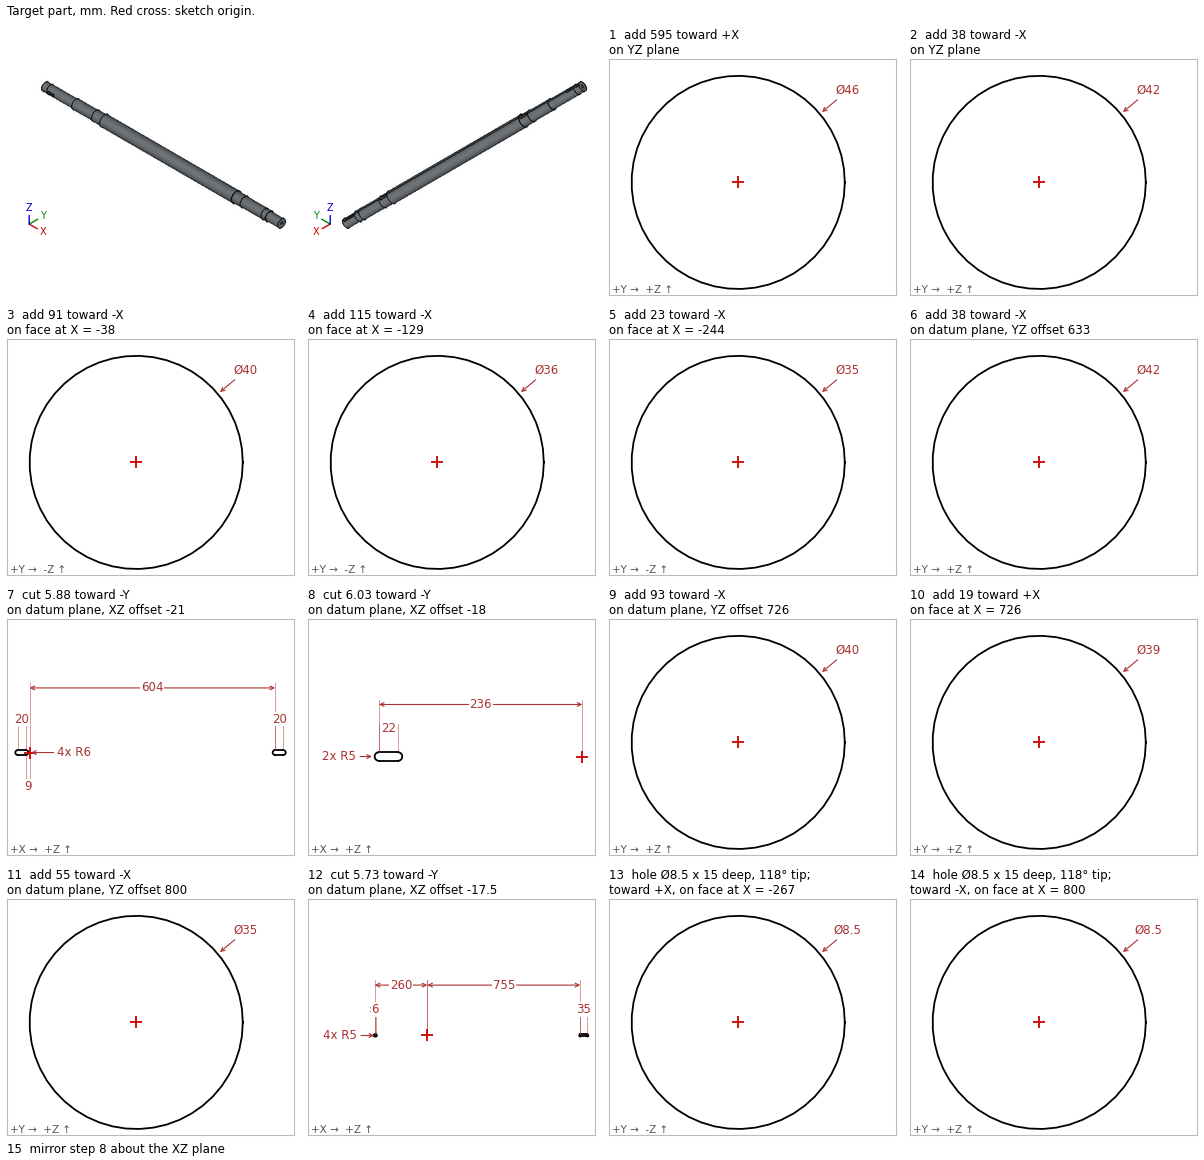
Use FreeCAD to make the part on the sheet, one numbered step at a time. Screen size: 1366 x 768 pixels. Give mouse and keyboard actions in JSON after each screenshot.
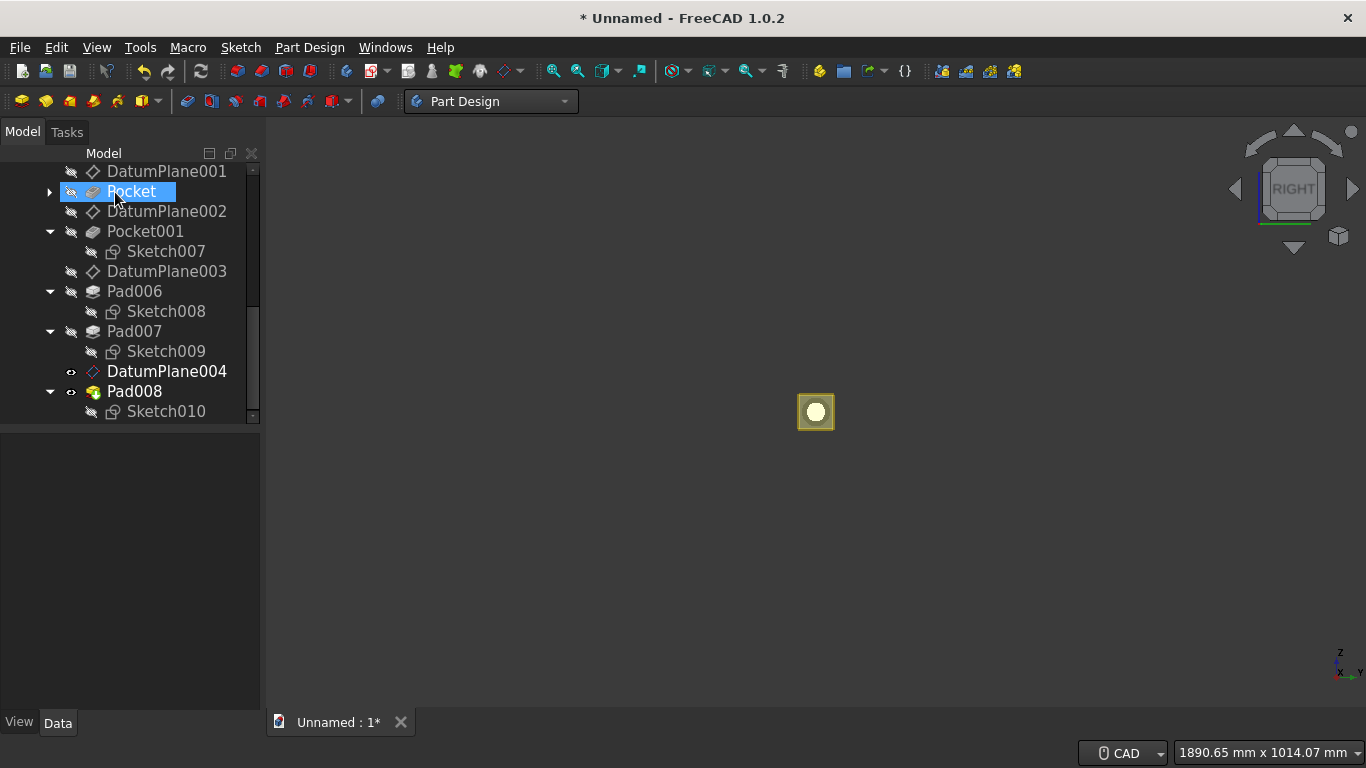
{"action": "left_click", "coordinate": [116, 372]}
{"action": "key", "text": "space"}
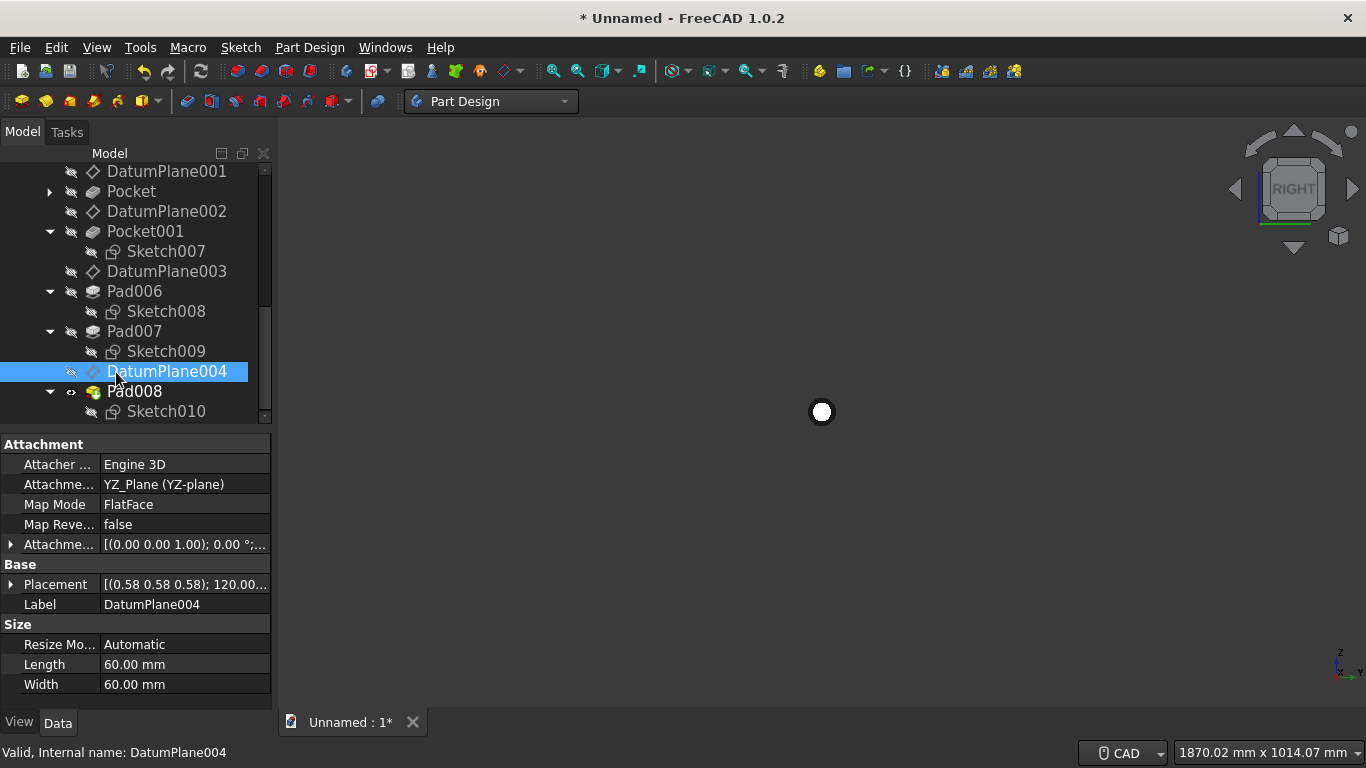
{"action": "key", "text": "v f"}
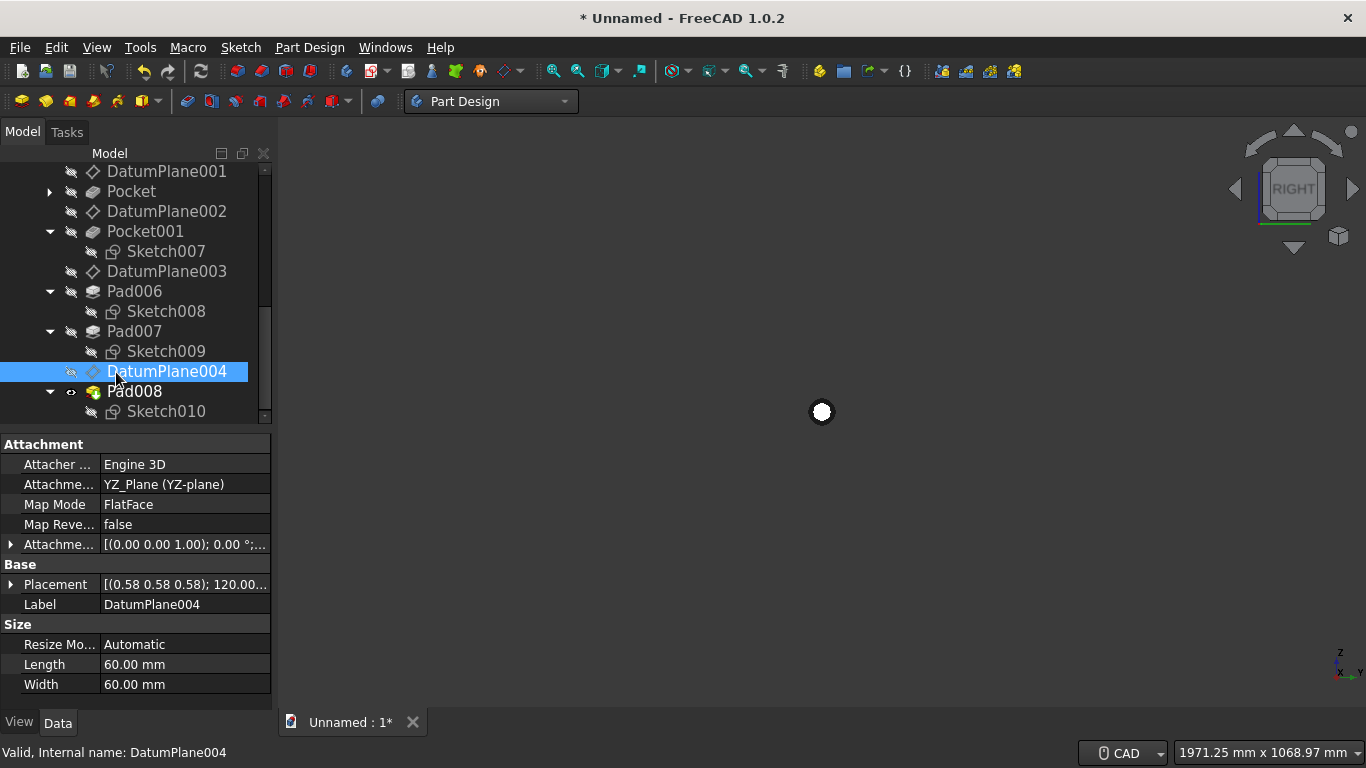
{"action": "scroll", "coordinate": [140, 287], "scroll_direction": "down", "scroll_amount": 3}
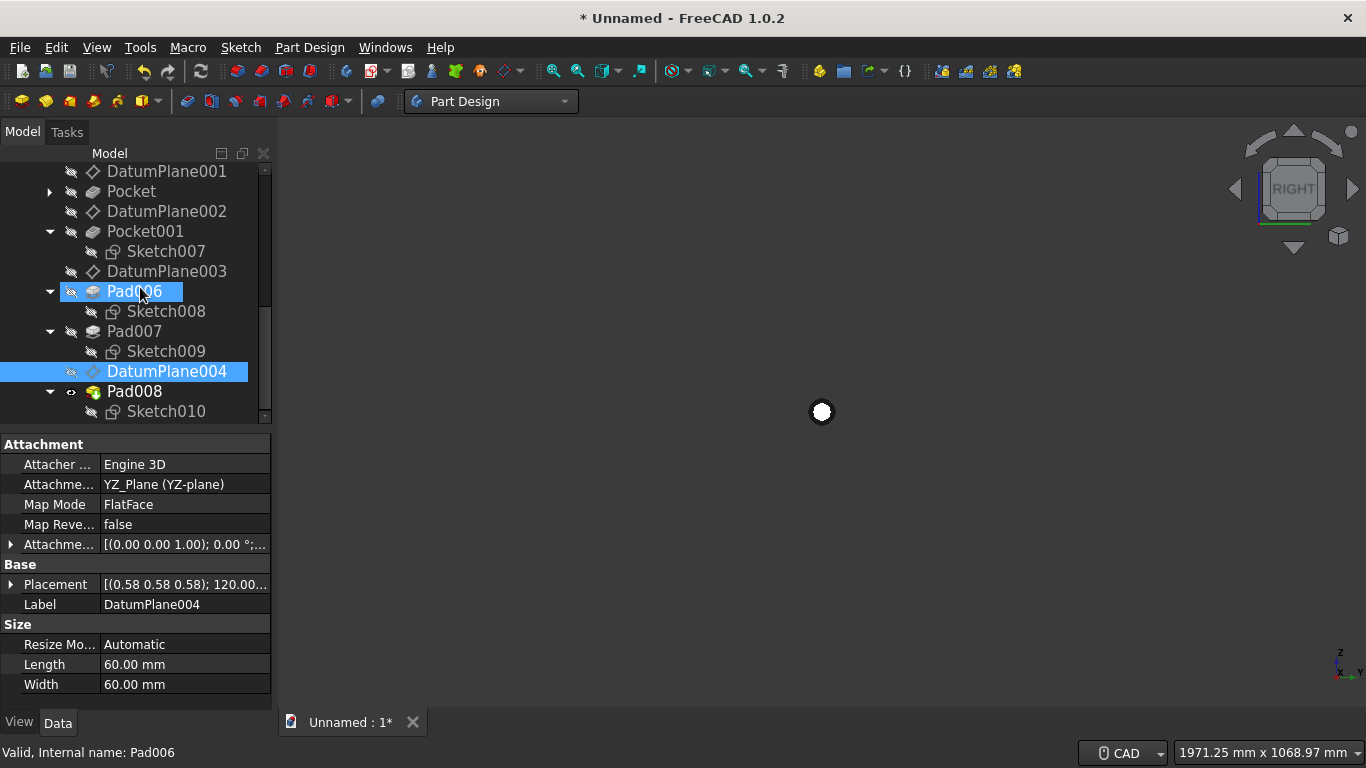
{"action": "scroll", "coordinate": [140, 287], "scroll_direction": "up", "scroll_amount": 15}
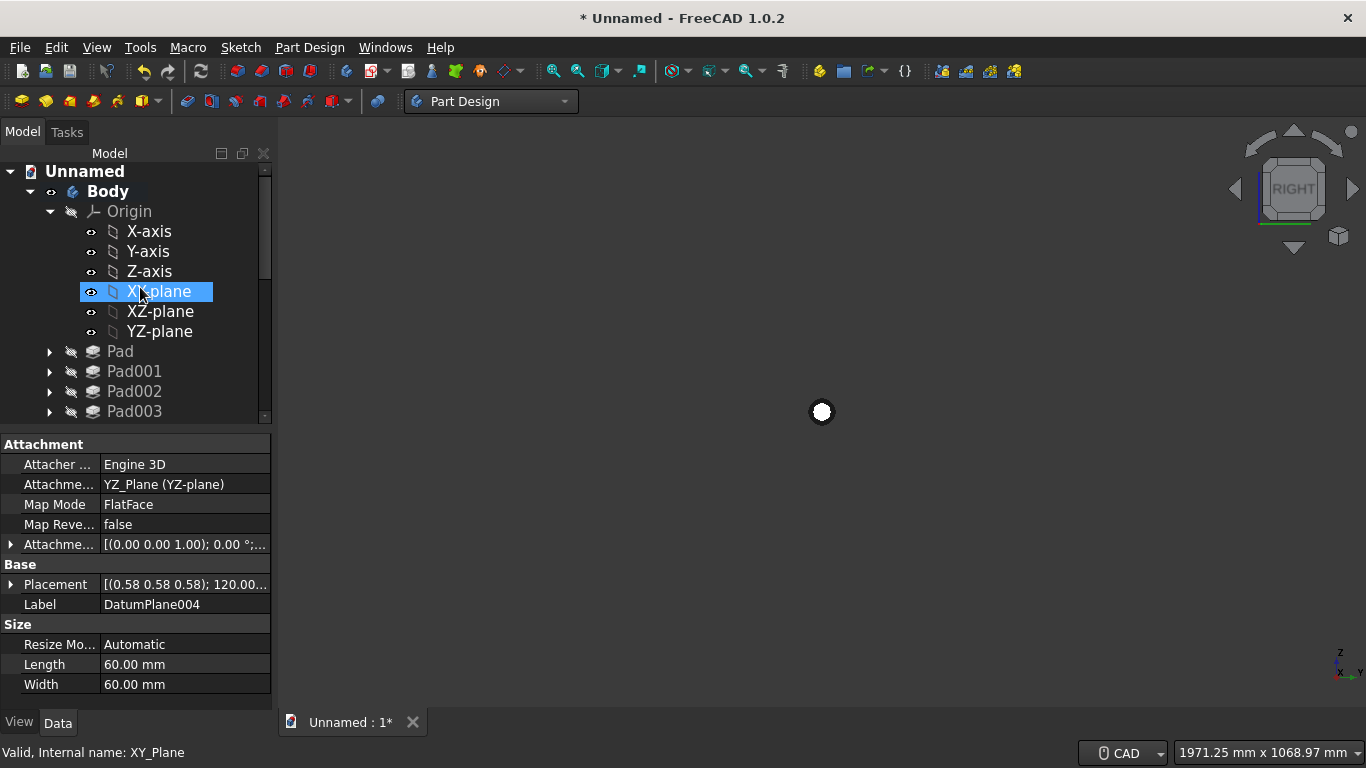
{"action": "left_click", "coordinate": [136, 312]}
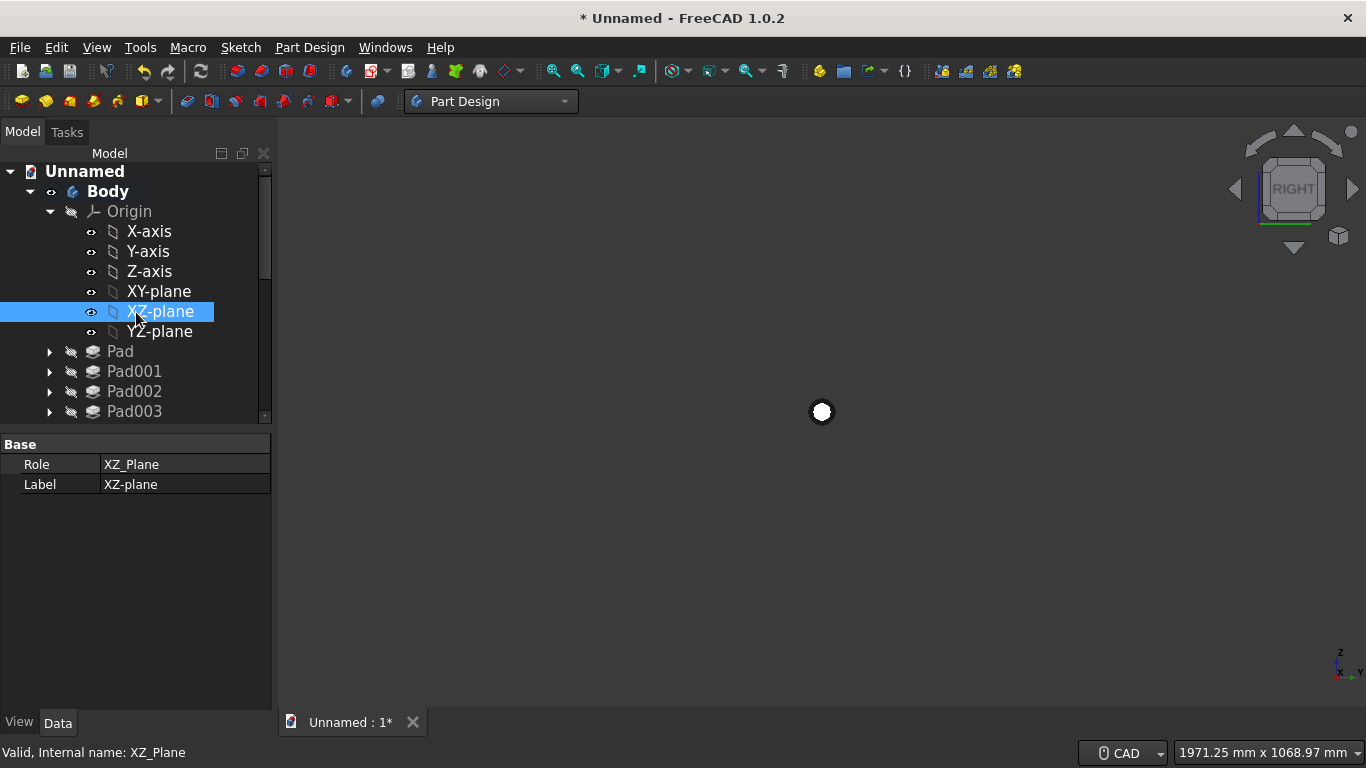
{"action": "left_click", "coordinate": [504, 72]}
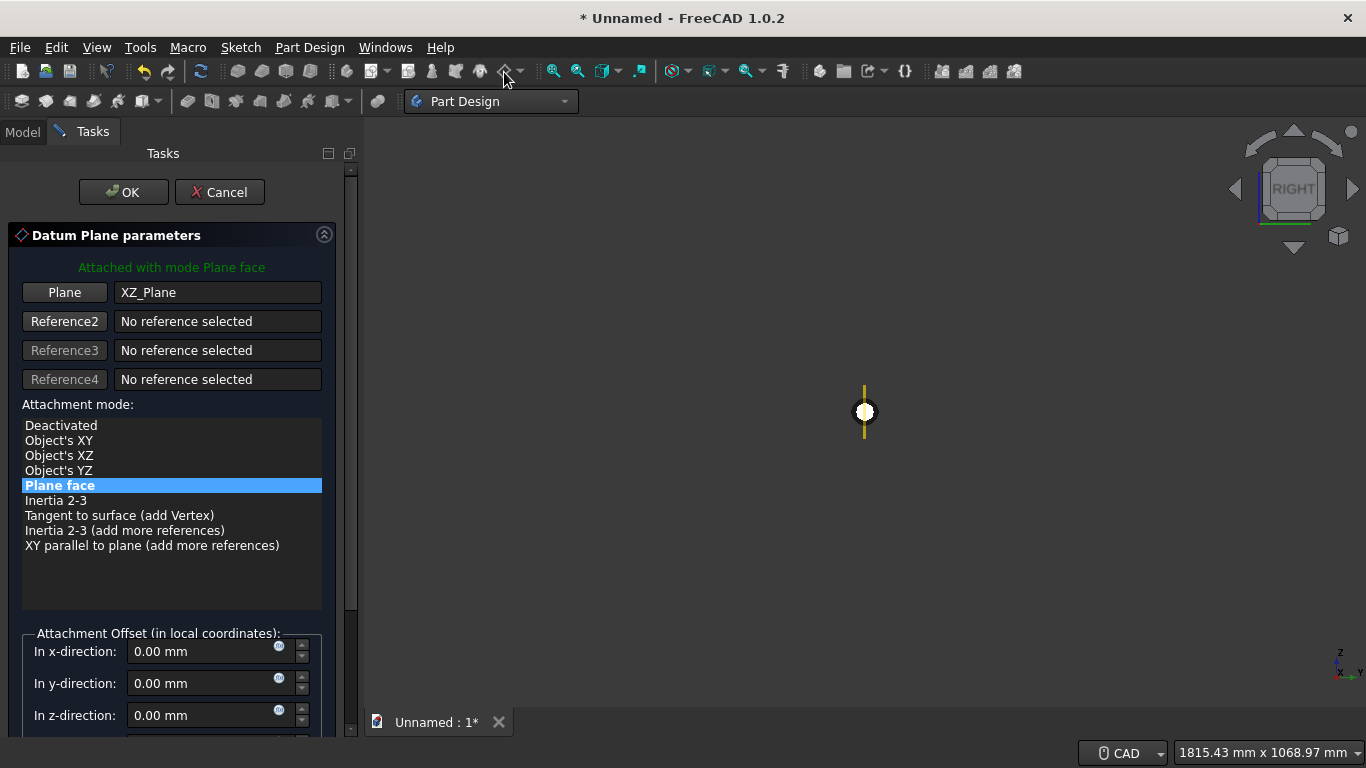
{"action": "triple_click", "coordinate": [210, 715]}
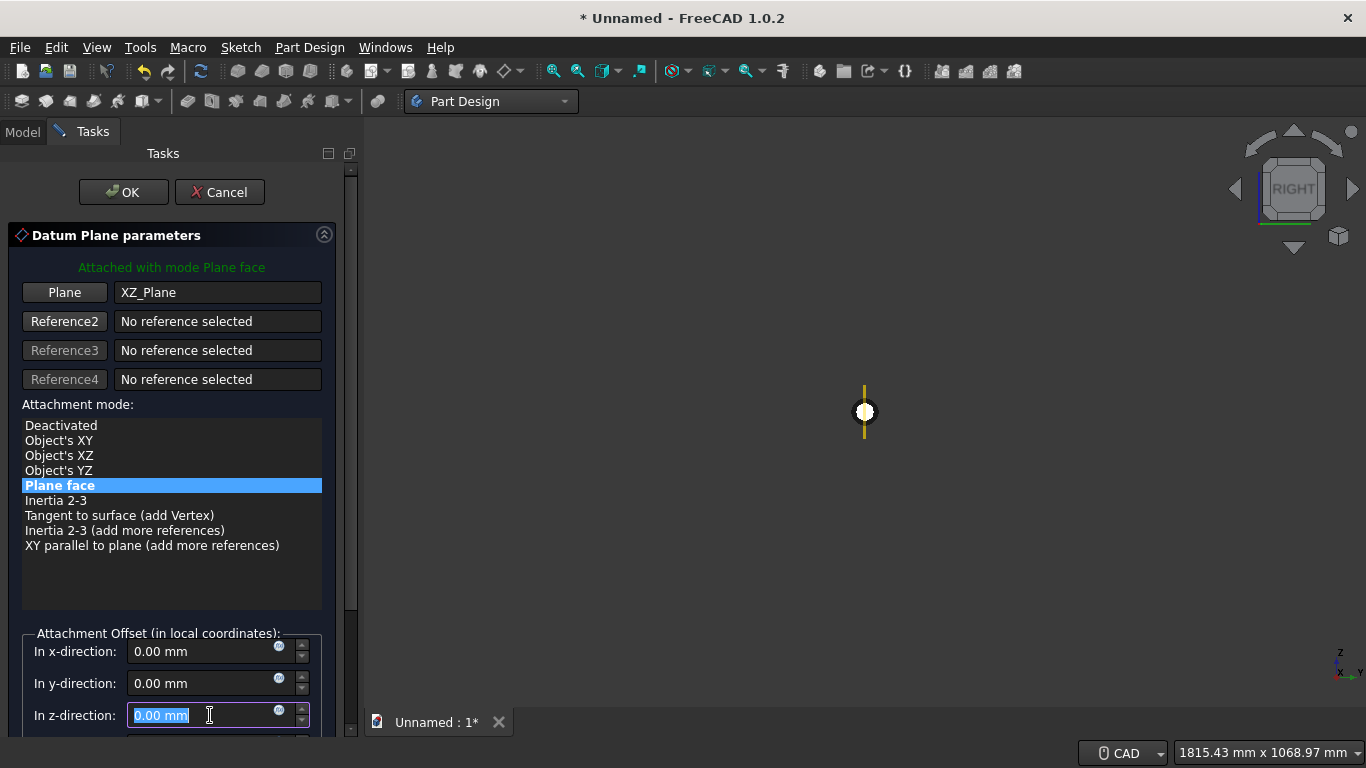
{"action": "type", "text": "-17.5"}
{"action": "key", "text": "Tab"}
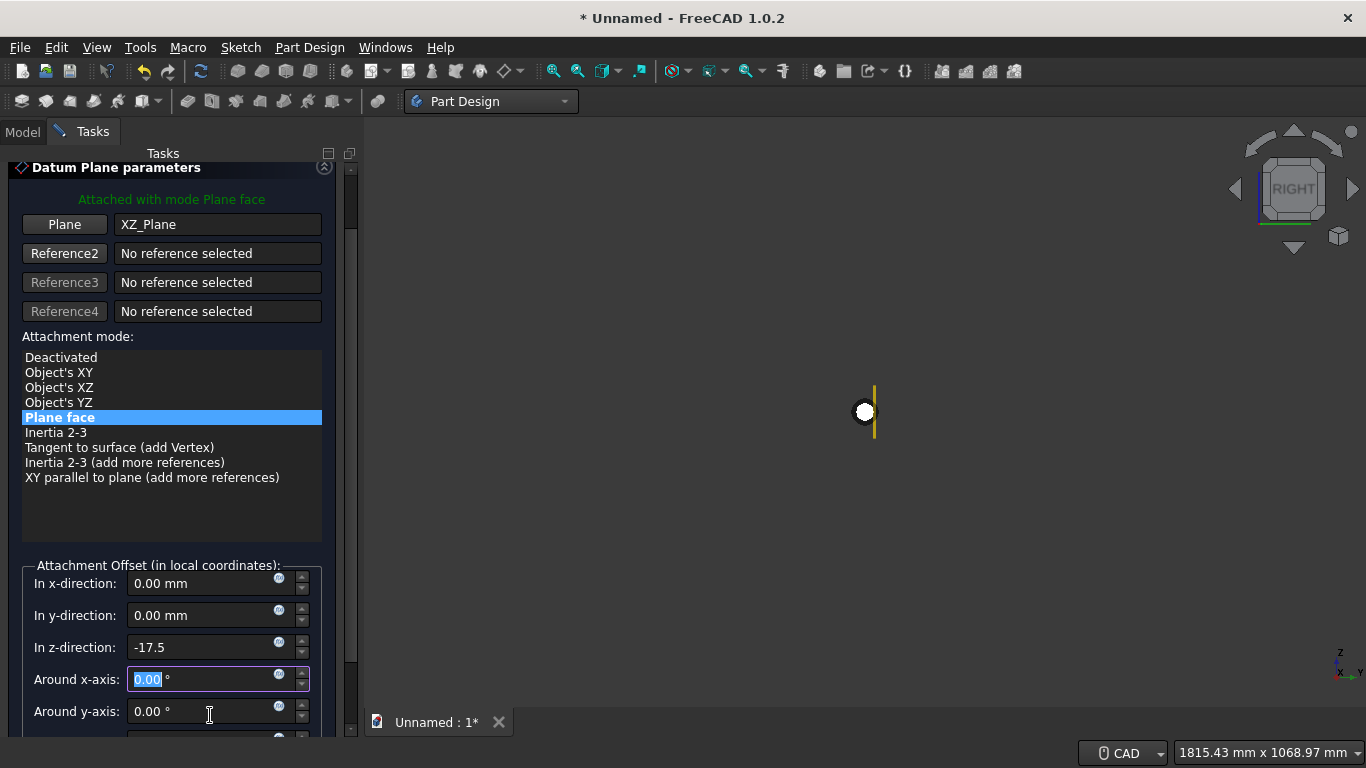
{"action": "scroll", "coordinate": [351, 450], "scroll_direction": "up", "scroll_amount": 2}